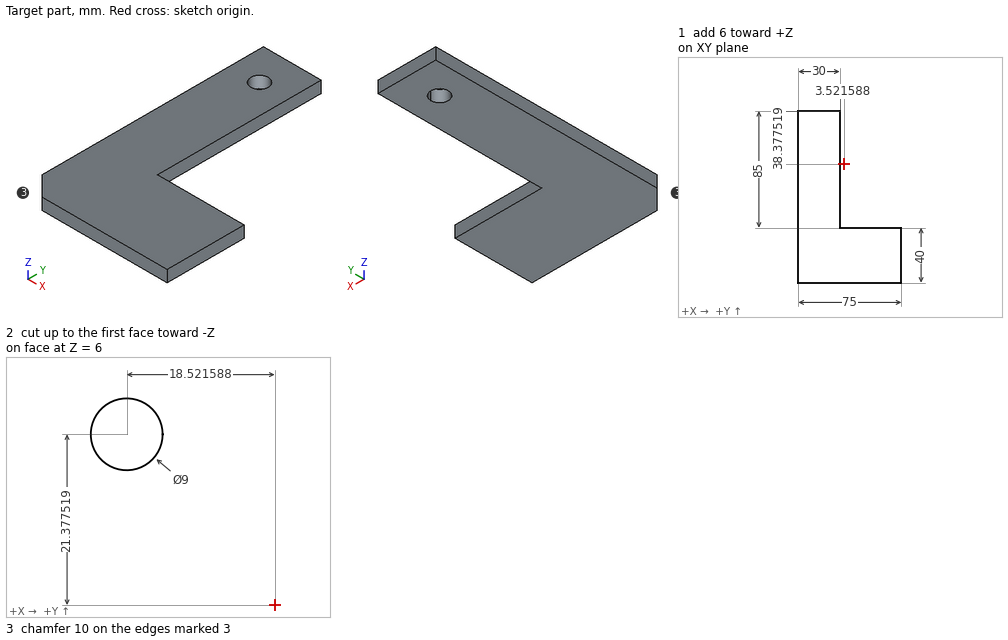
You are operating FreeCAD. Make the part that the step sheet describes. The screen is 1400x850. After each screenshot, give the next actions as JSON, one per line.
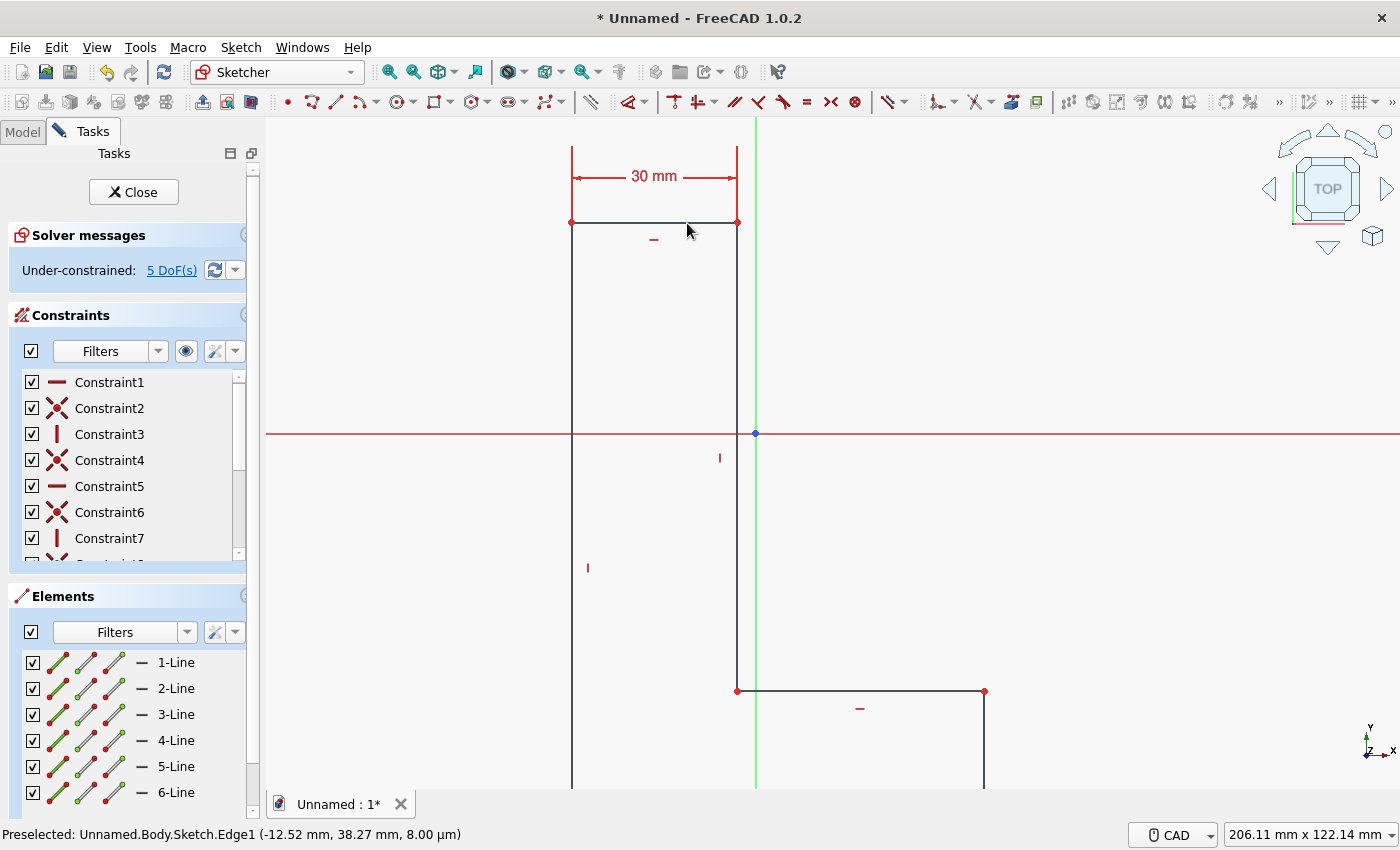
{"action": "scroll", "coordinate": [737, 223], "scroll_direction": "down", "scroll_amount": 2}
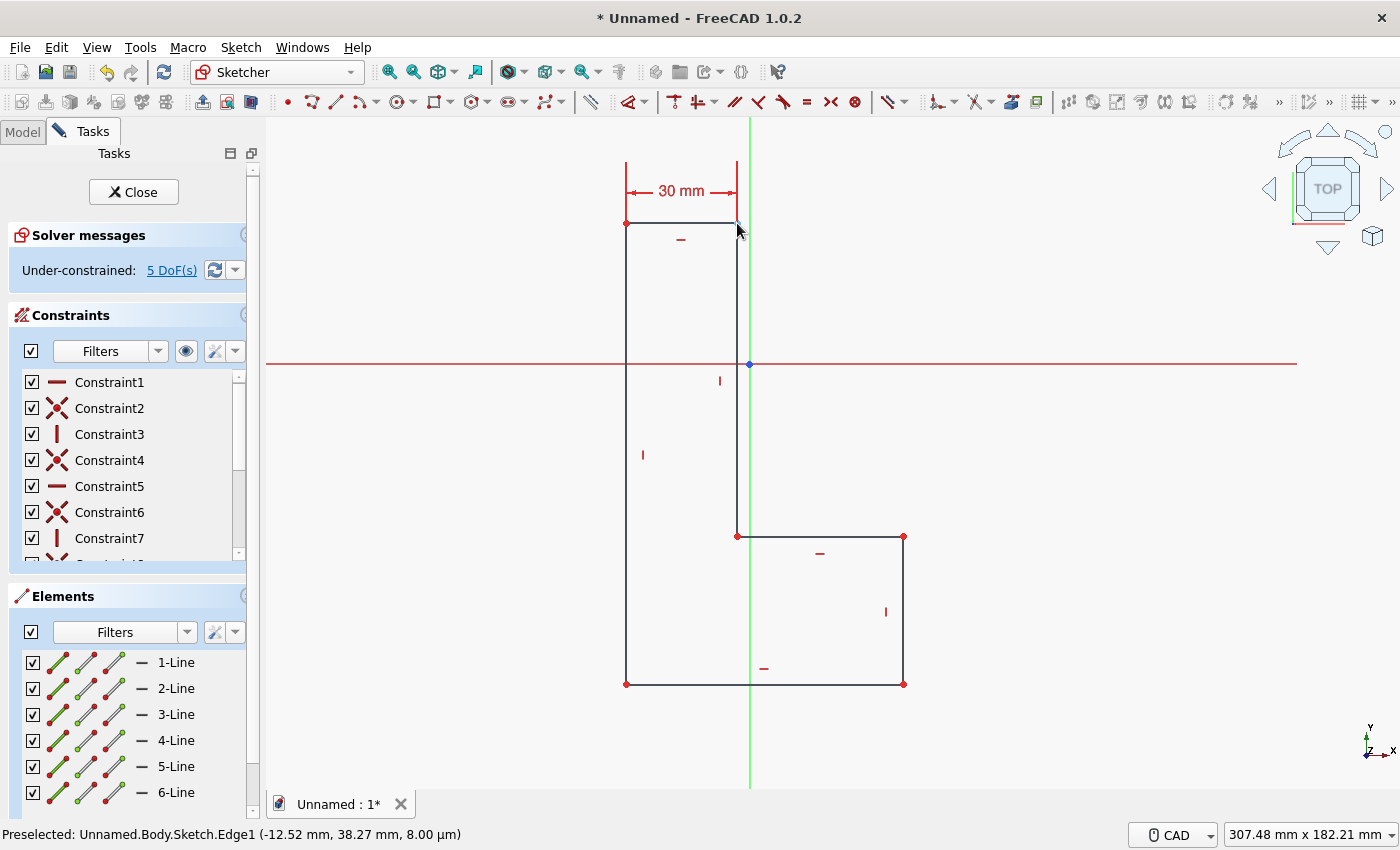
{"action": "left_click", "coordinate": [709, 685]}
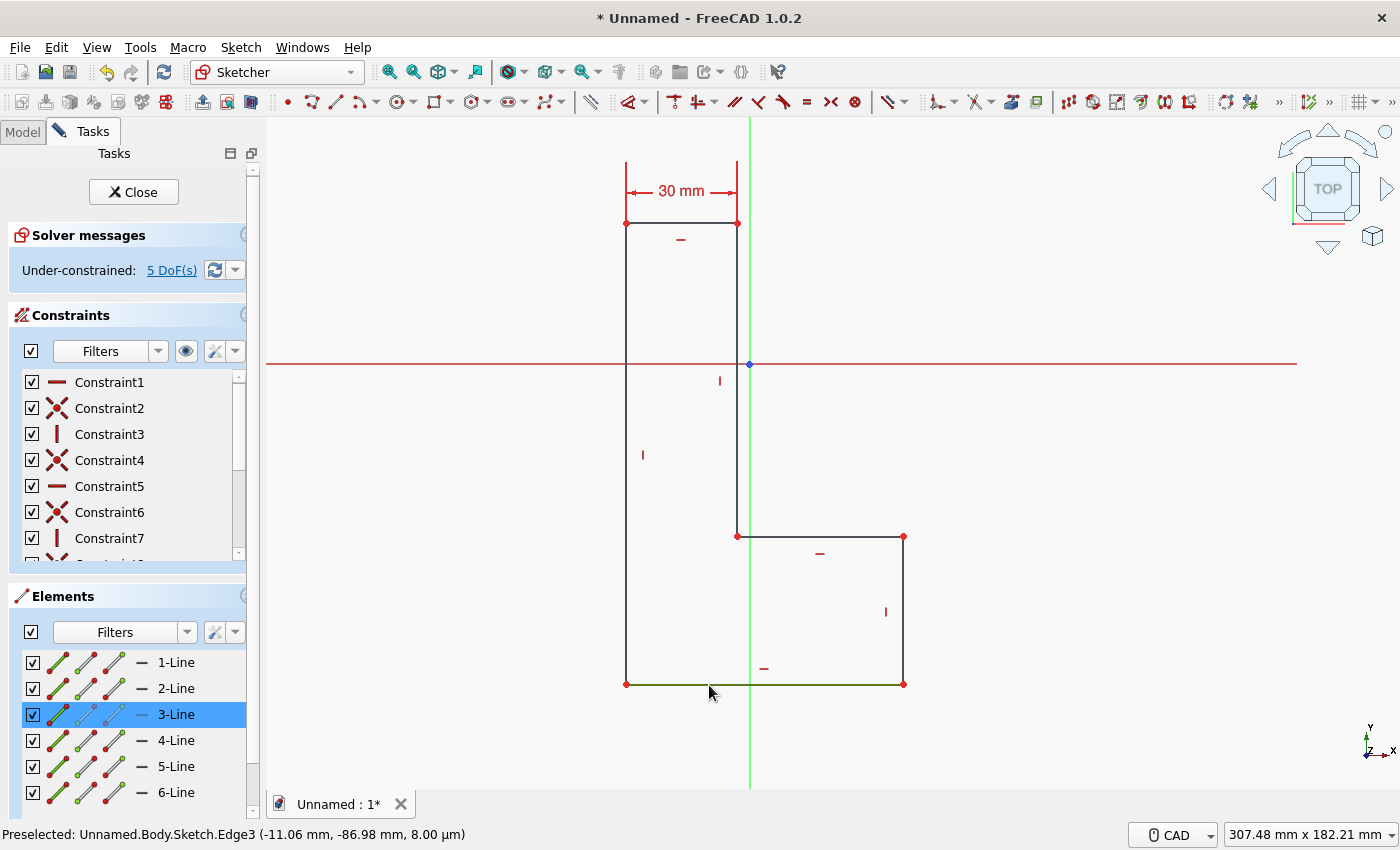
{"action": "key", "text": "l"}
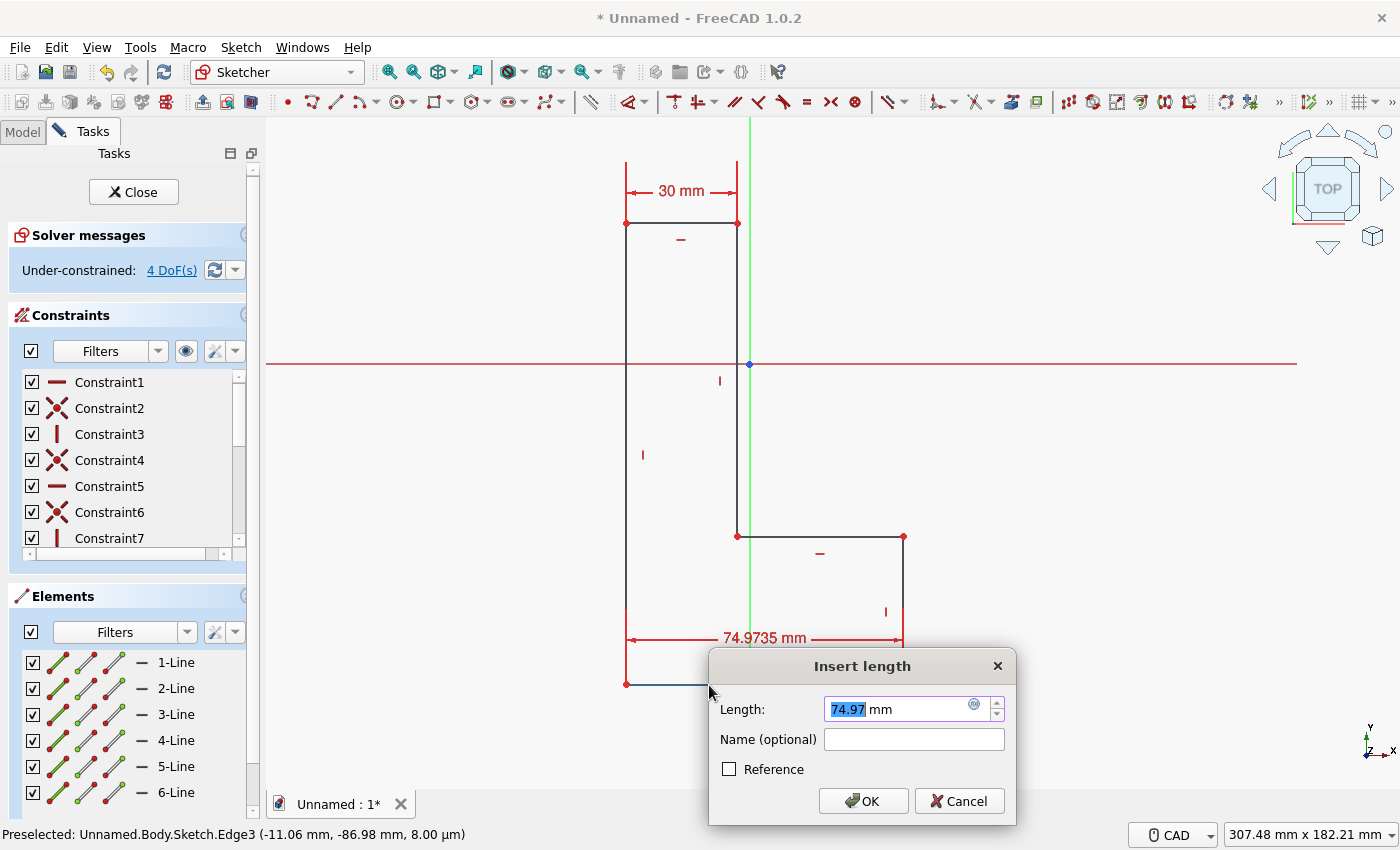
{"action": "type", "text": "75"}
{"action": "key", "text": "Return"}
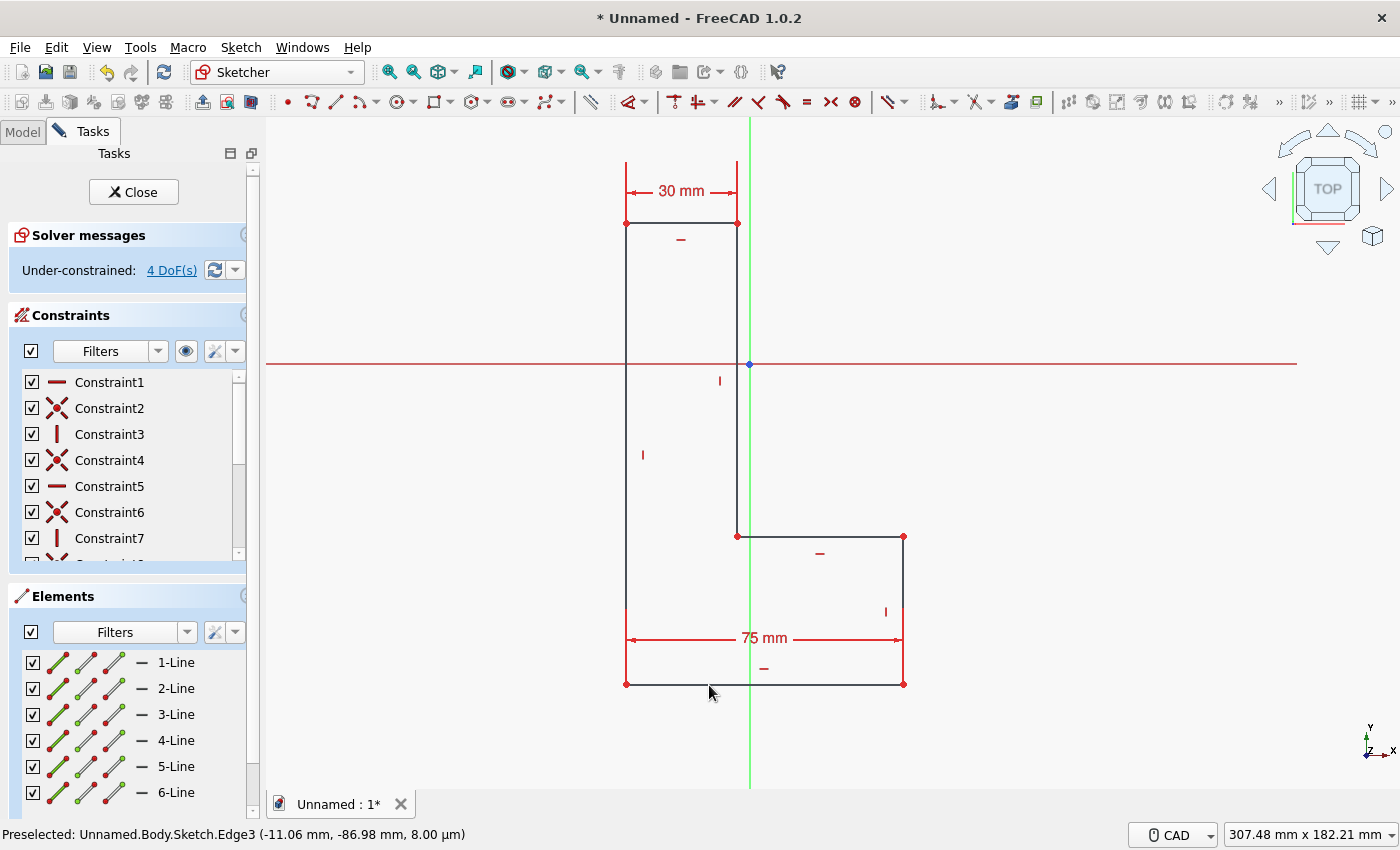
{"action": "left_click", "coordinate": [903, 641]}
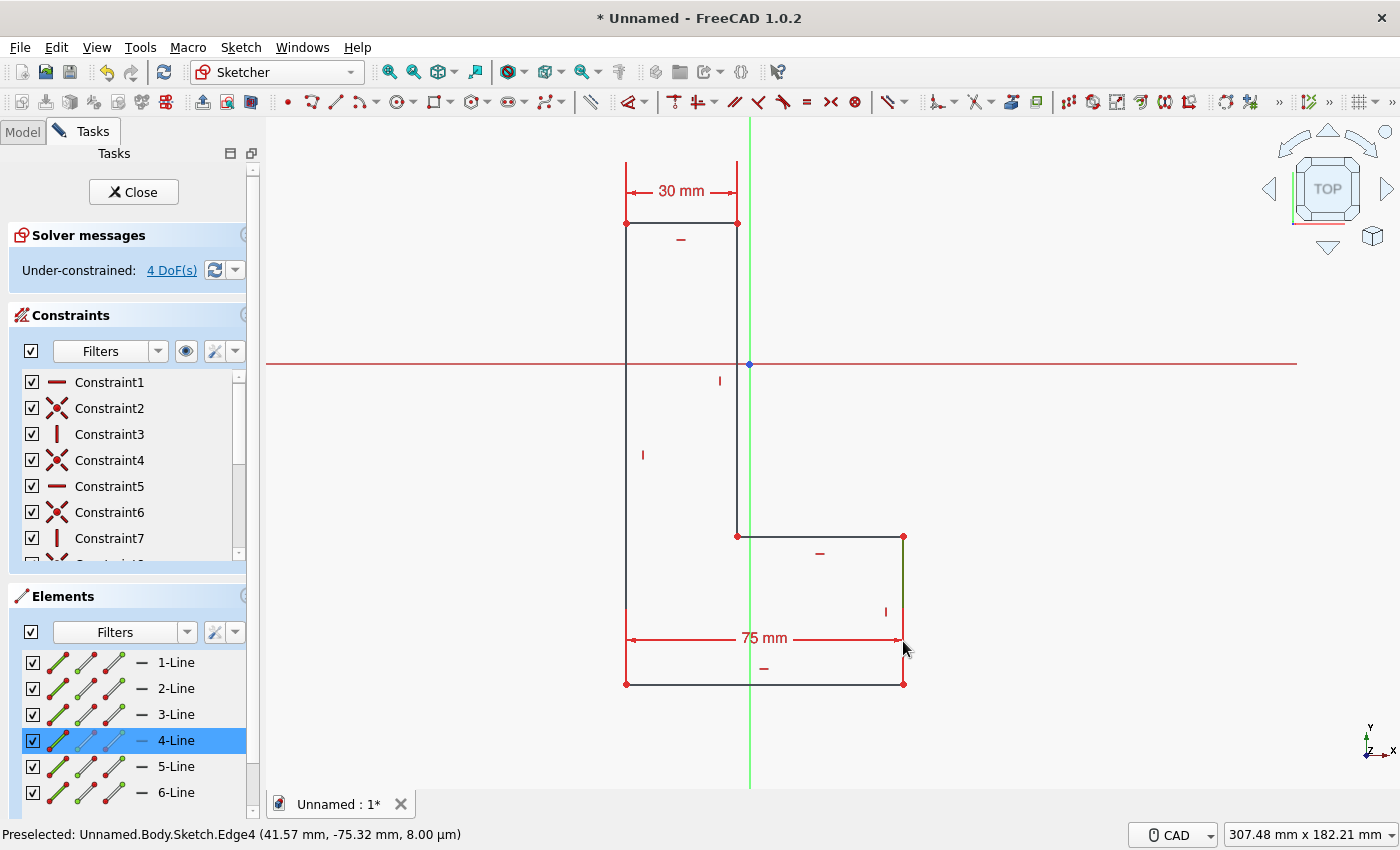
{"action": "key", "text": "i"}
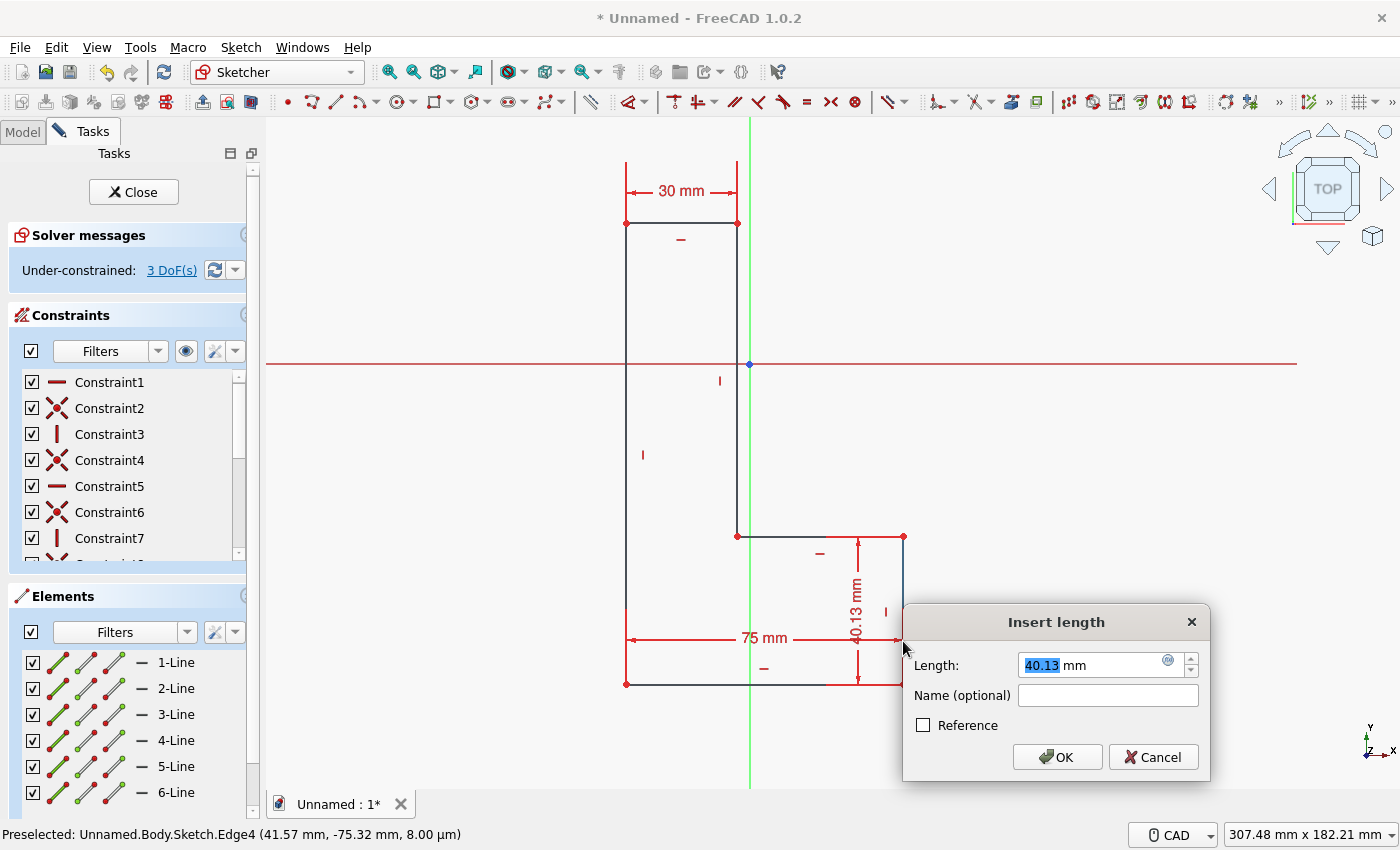
{"action": "type", "text": "40"}
{"action": "key", "text": "Return"}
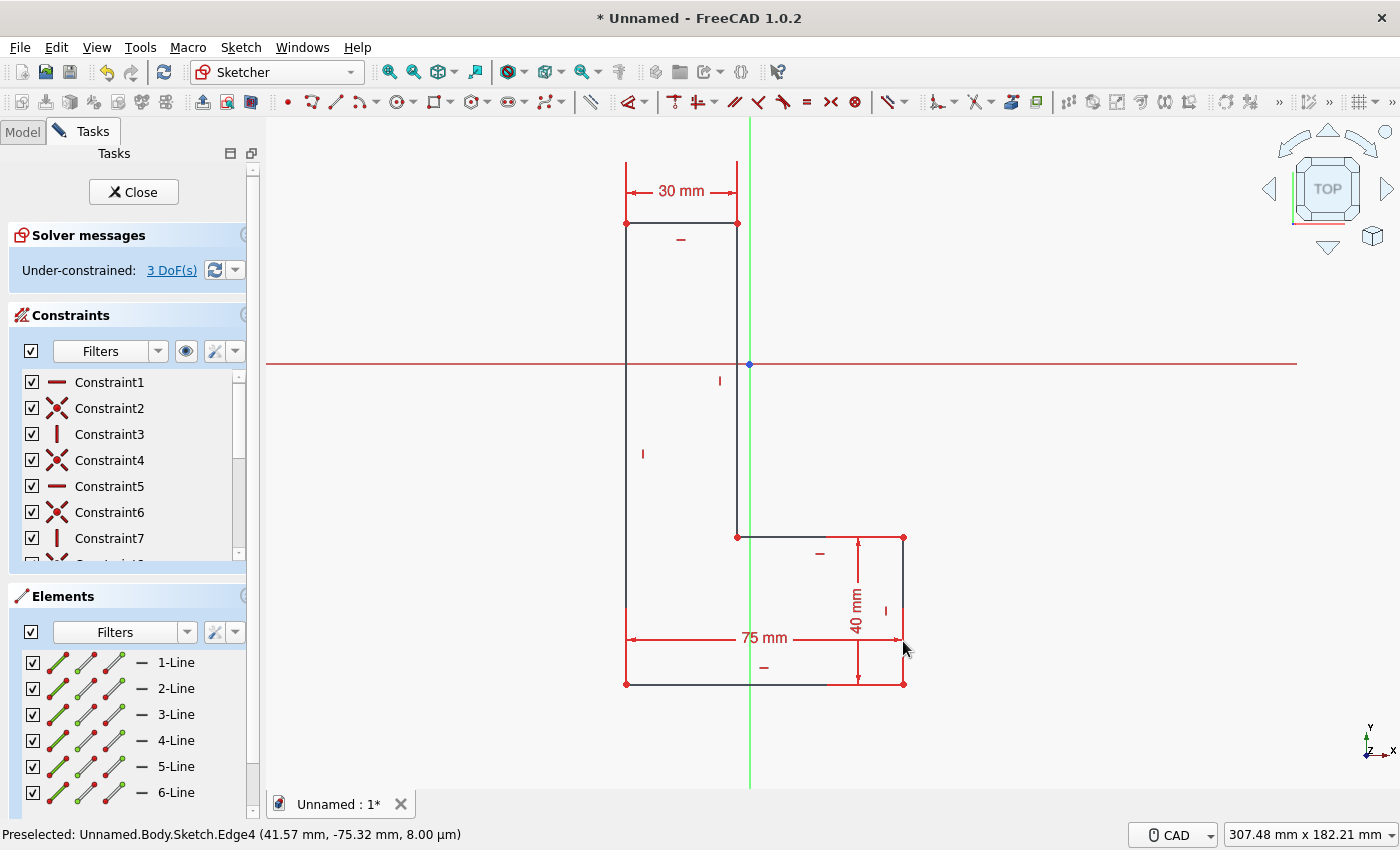
{"action": "left_click", "coordinate": [737, 443]}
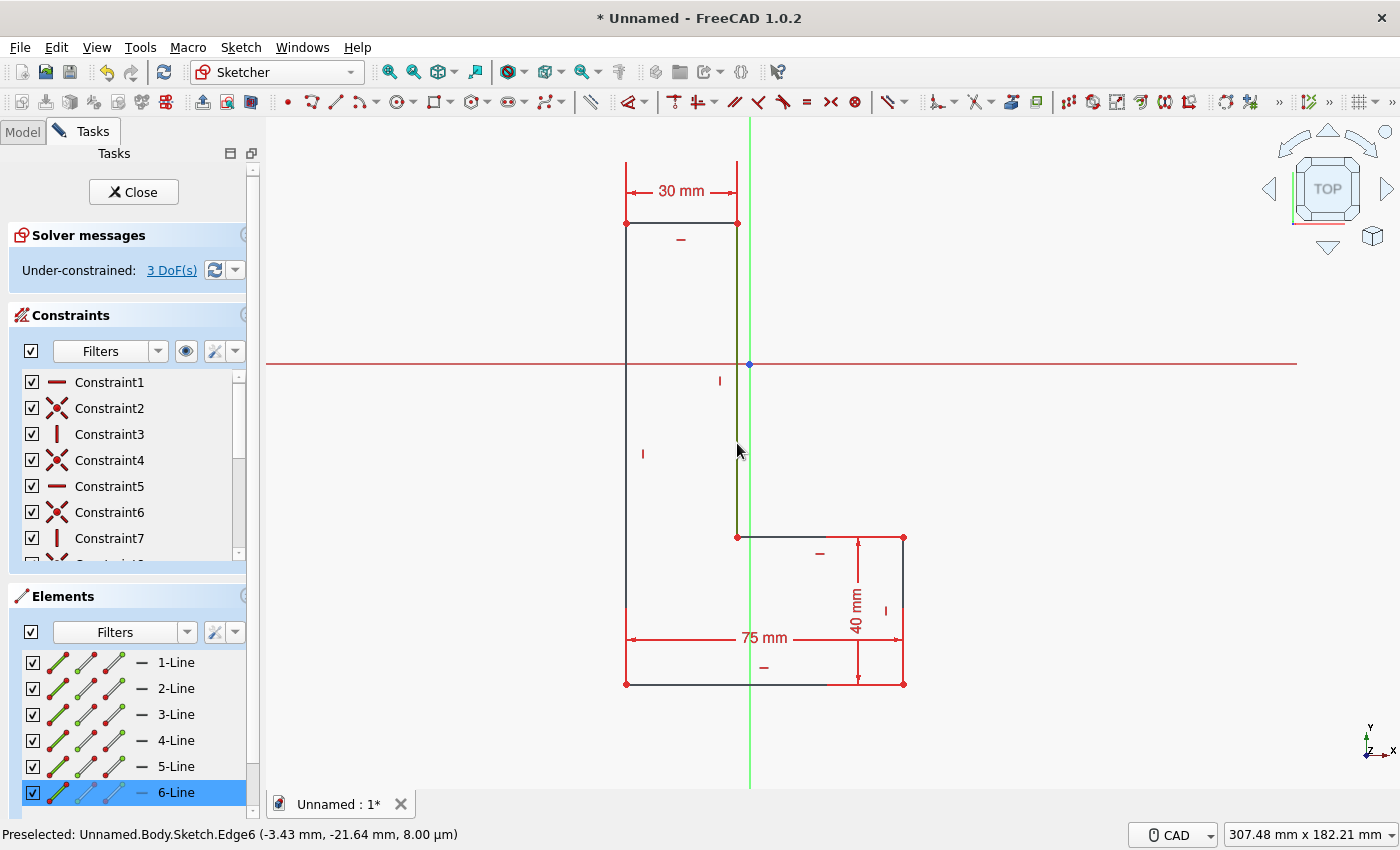
{"action": "left_click", "coordinate": [646, 102]}